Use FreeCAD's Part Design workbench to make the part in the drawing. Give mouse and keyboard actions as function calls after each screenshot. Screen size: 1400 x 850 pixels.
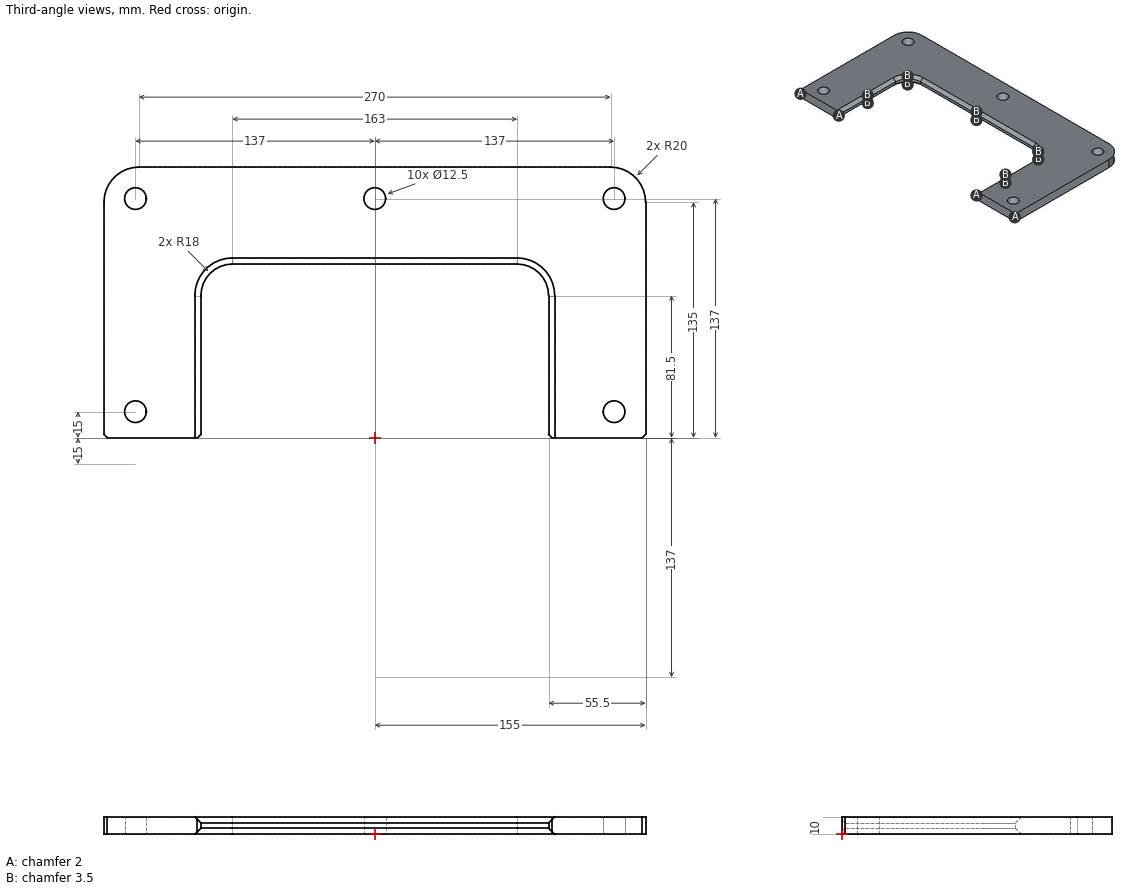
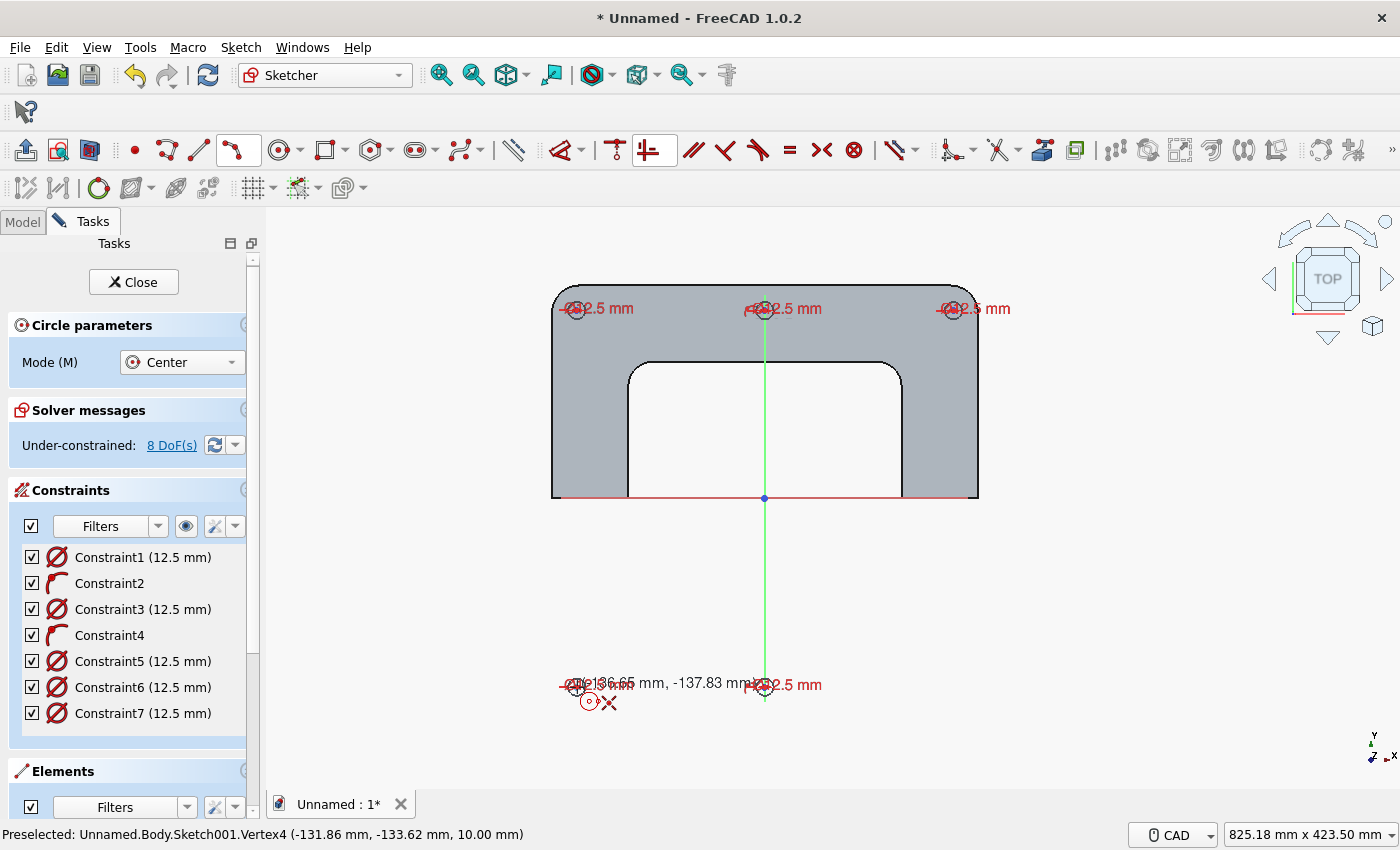
scroll(953, 687, up, 5)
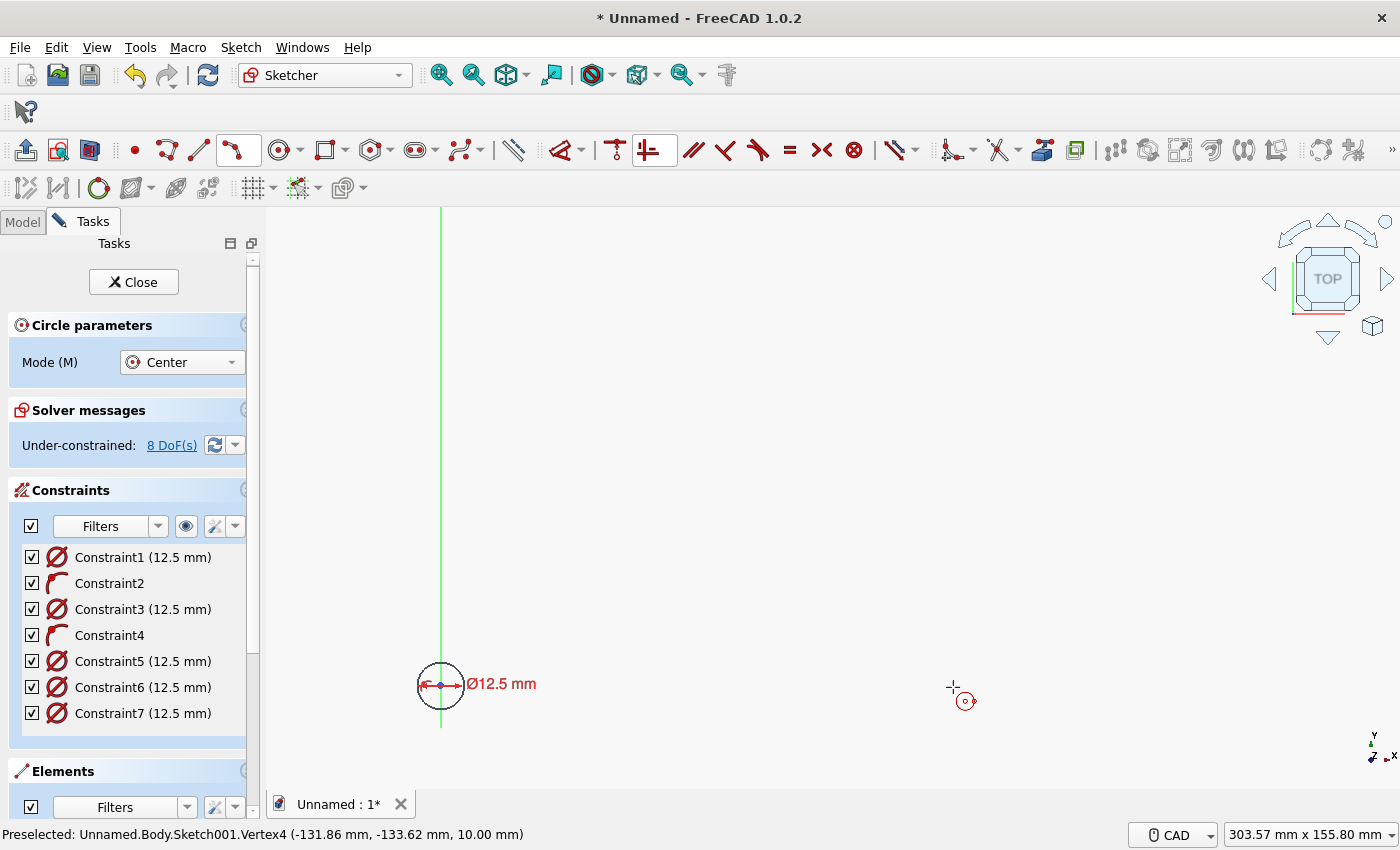
click(953, 685)
move(969, 668)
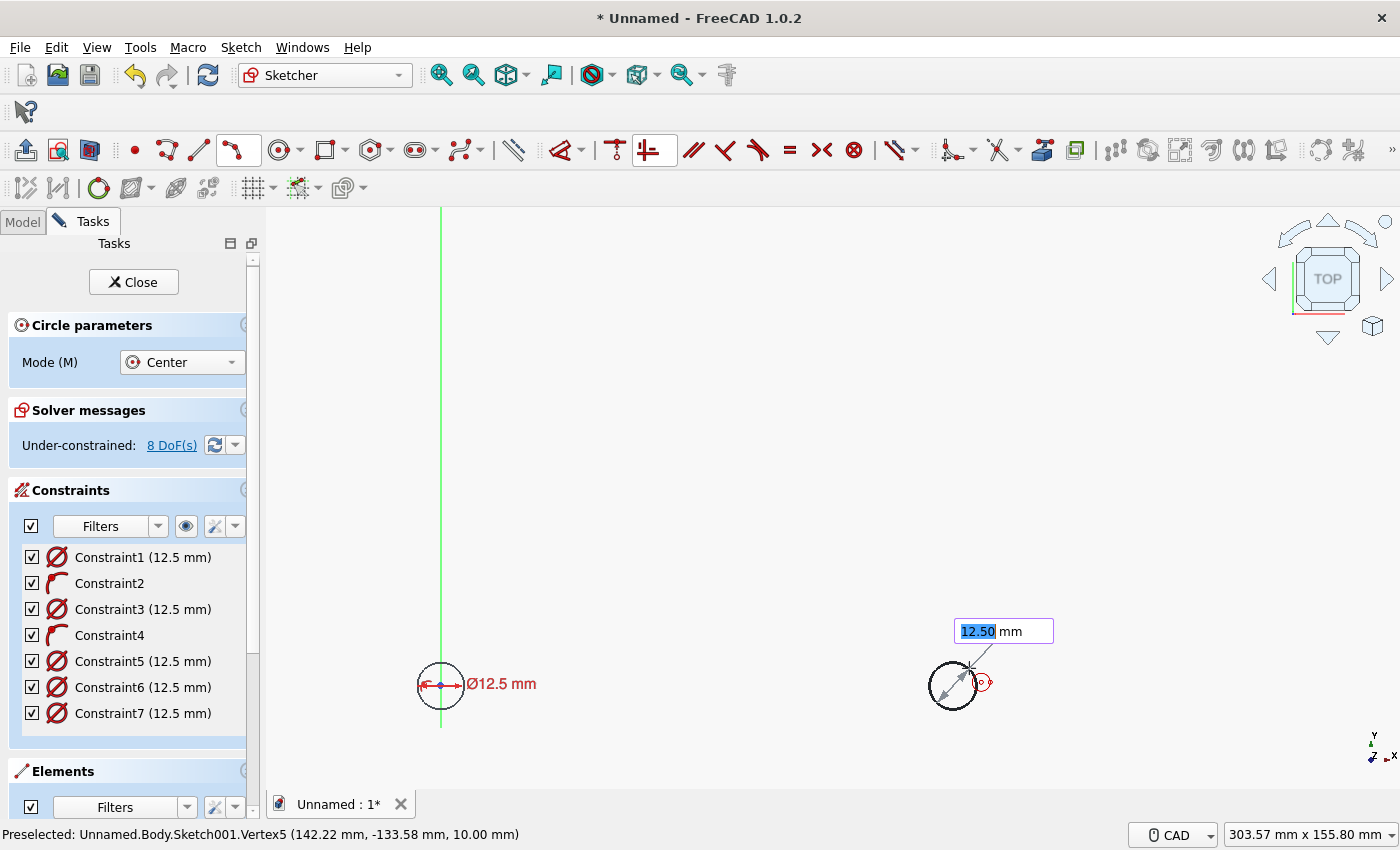
text(12.5)
key(Return)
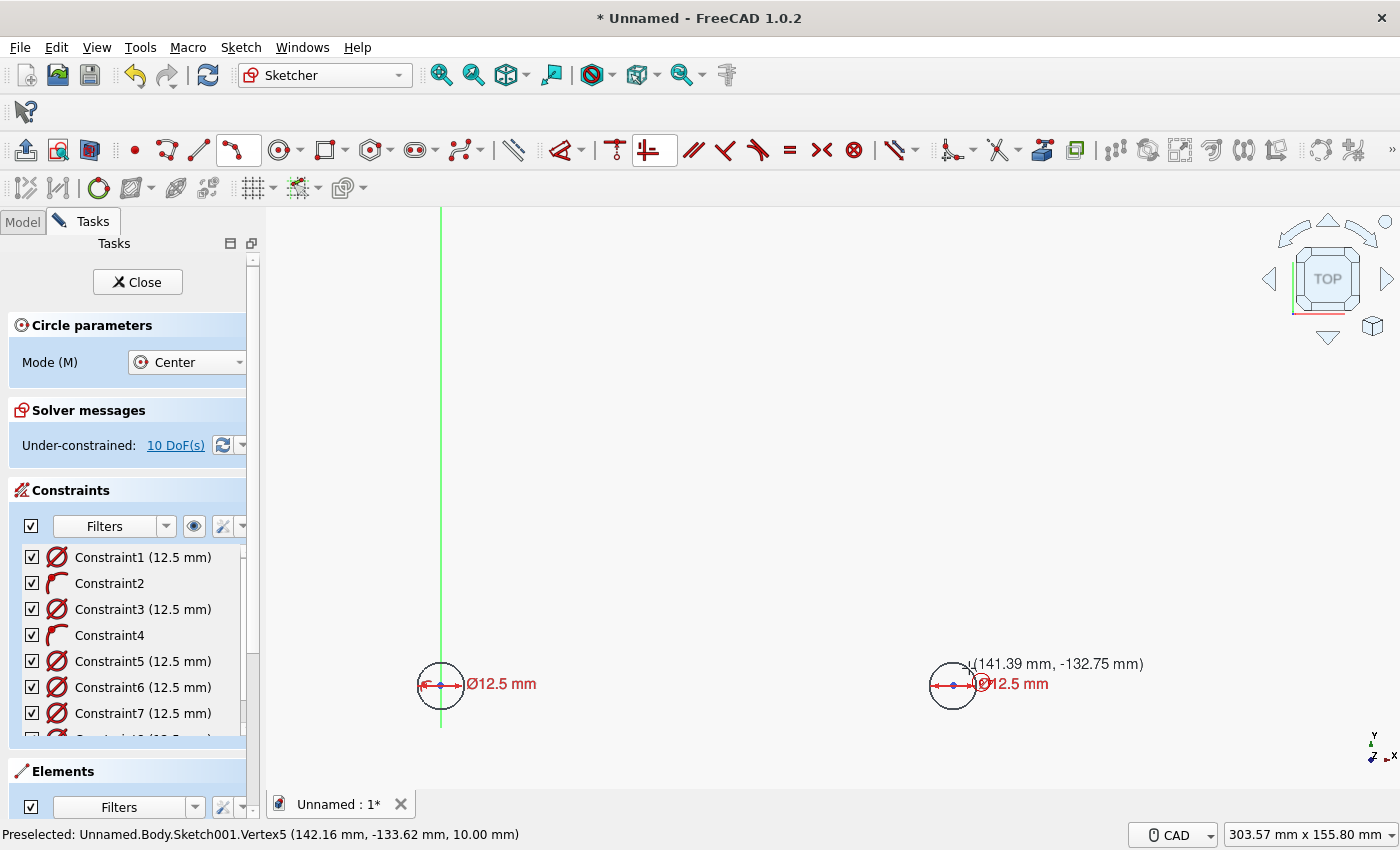
scroll(953, 687, down, 5)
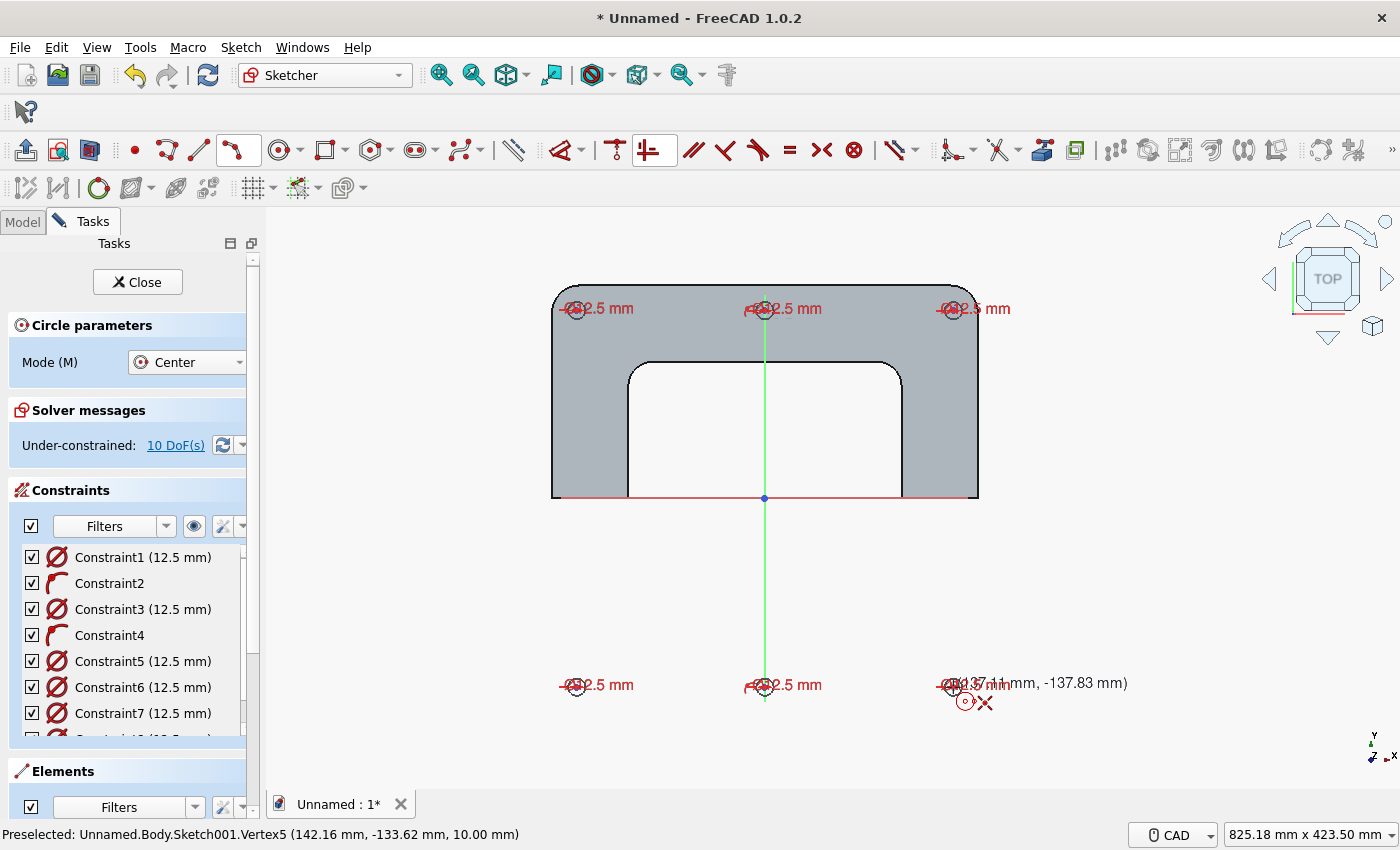
scroll(577, 478, up, 5)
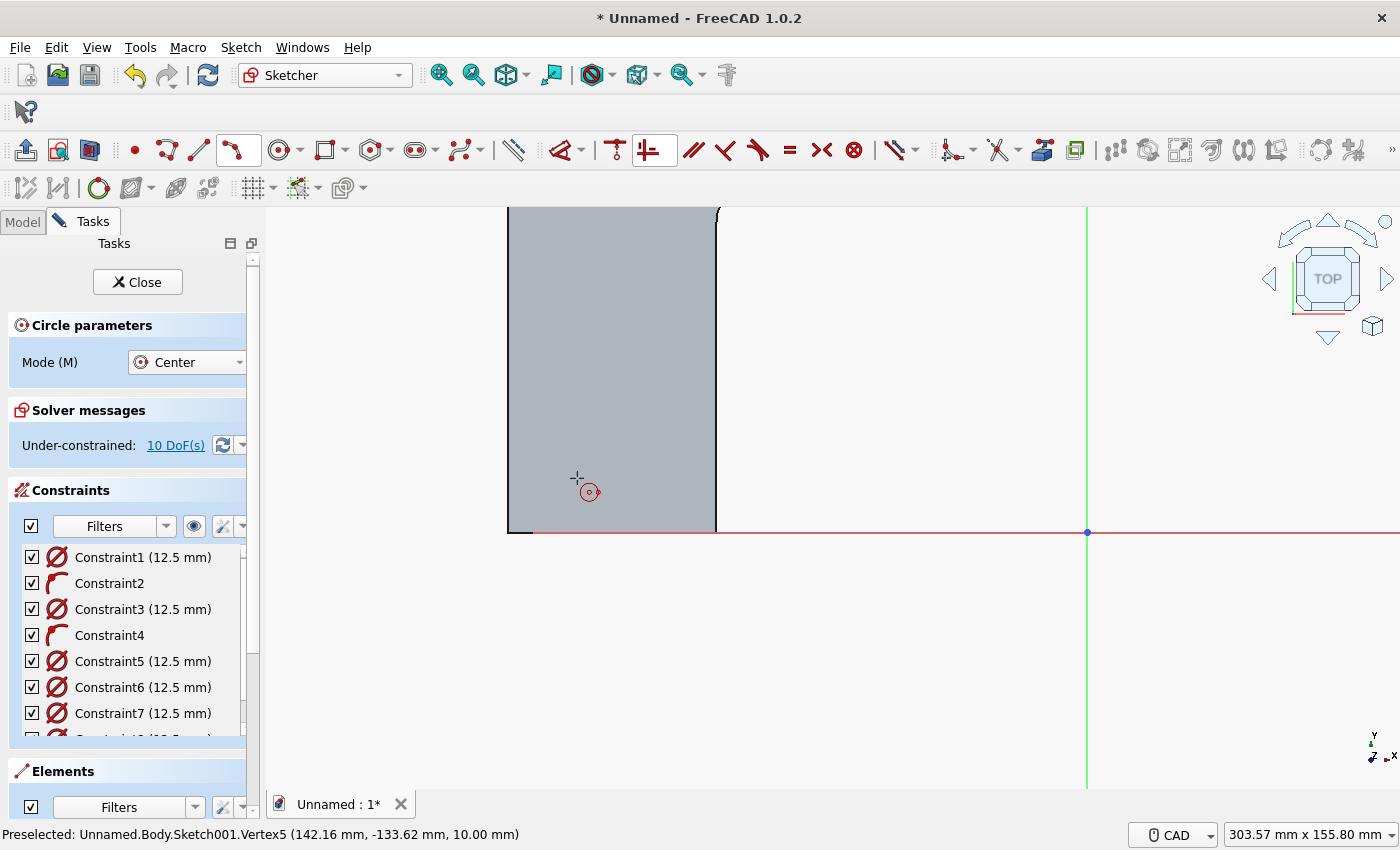
click(576, 477)
move(592, 460)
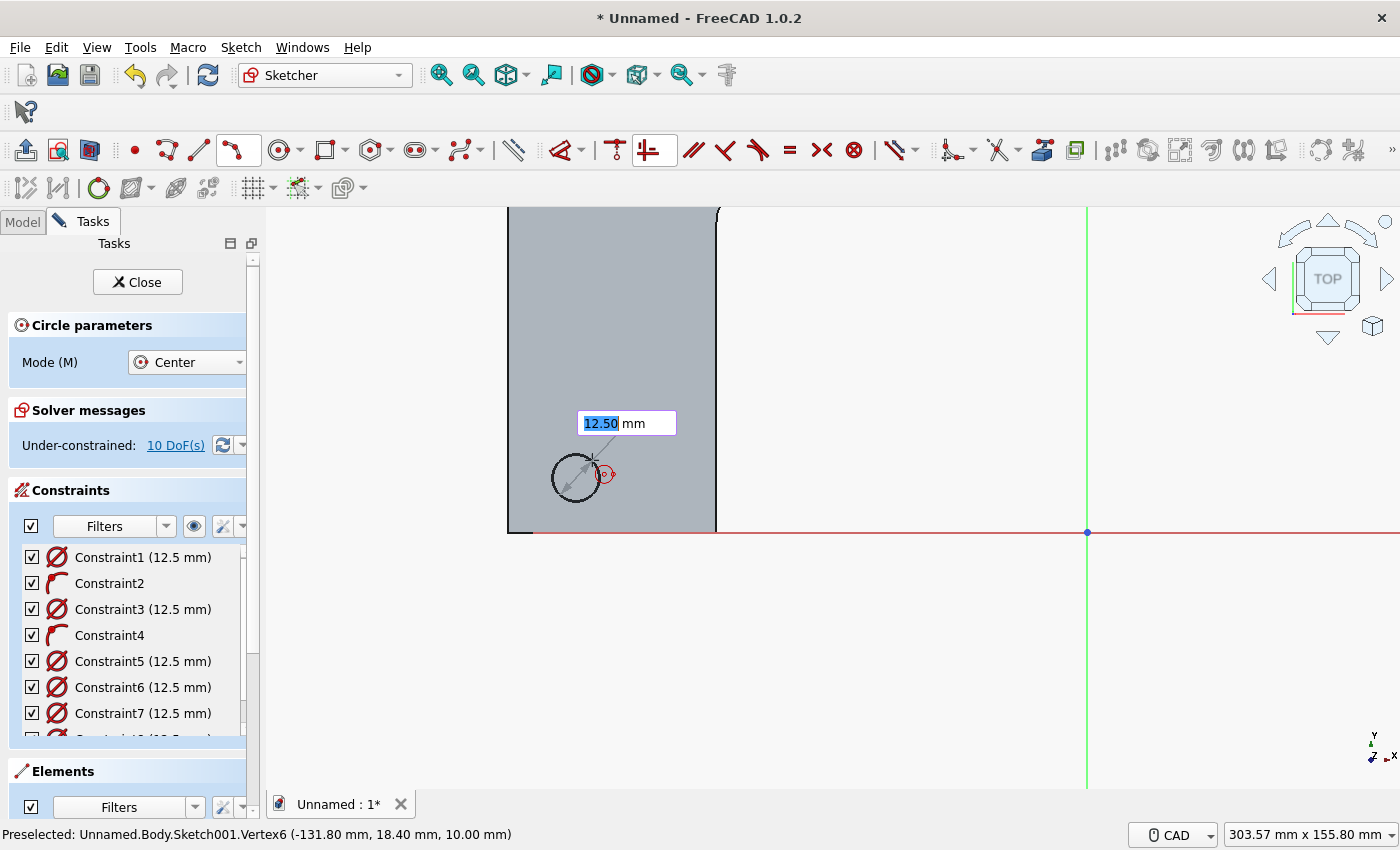
text(12.5)
key(Return)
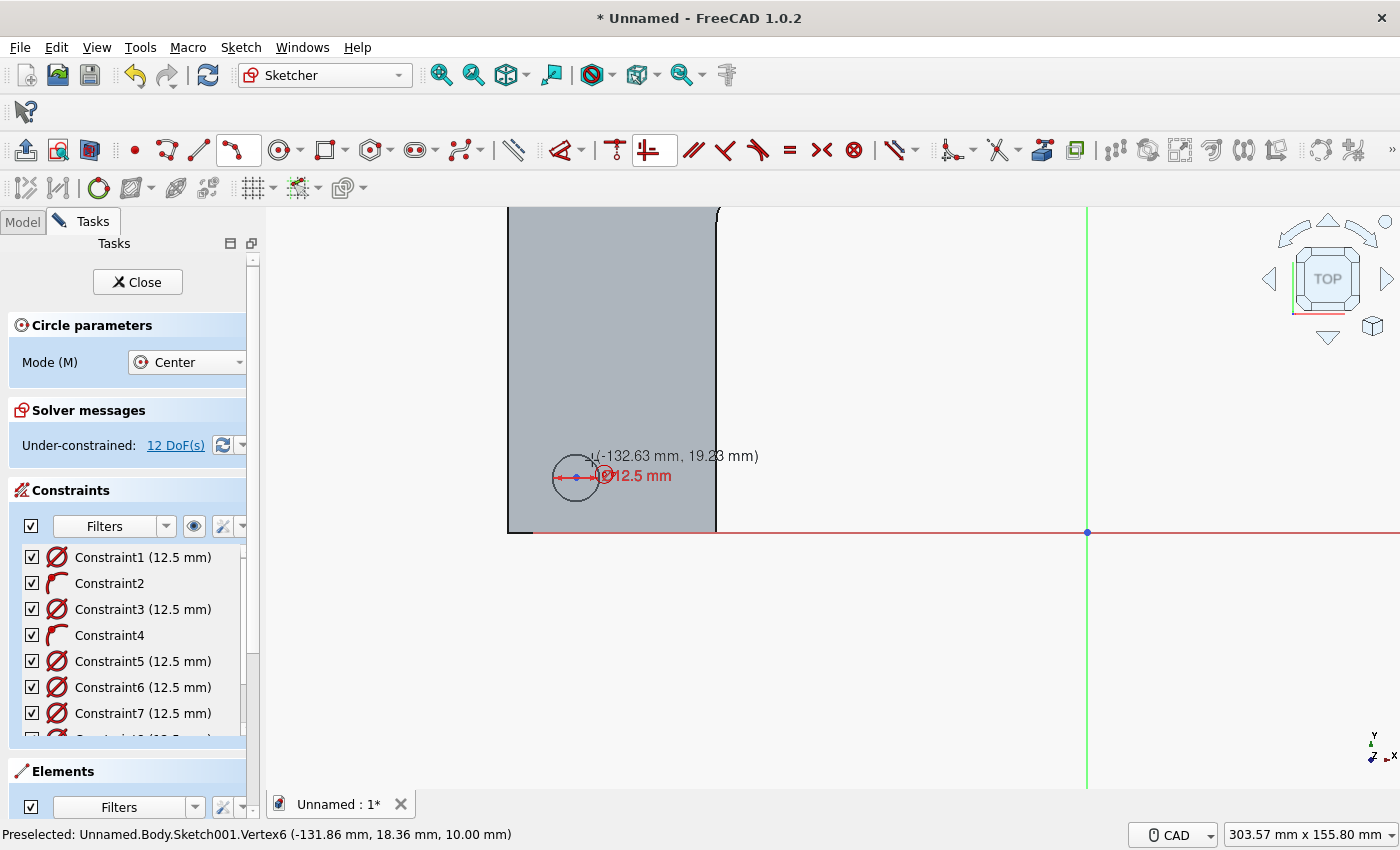
click(576, 589)
move(592, 572)